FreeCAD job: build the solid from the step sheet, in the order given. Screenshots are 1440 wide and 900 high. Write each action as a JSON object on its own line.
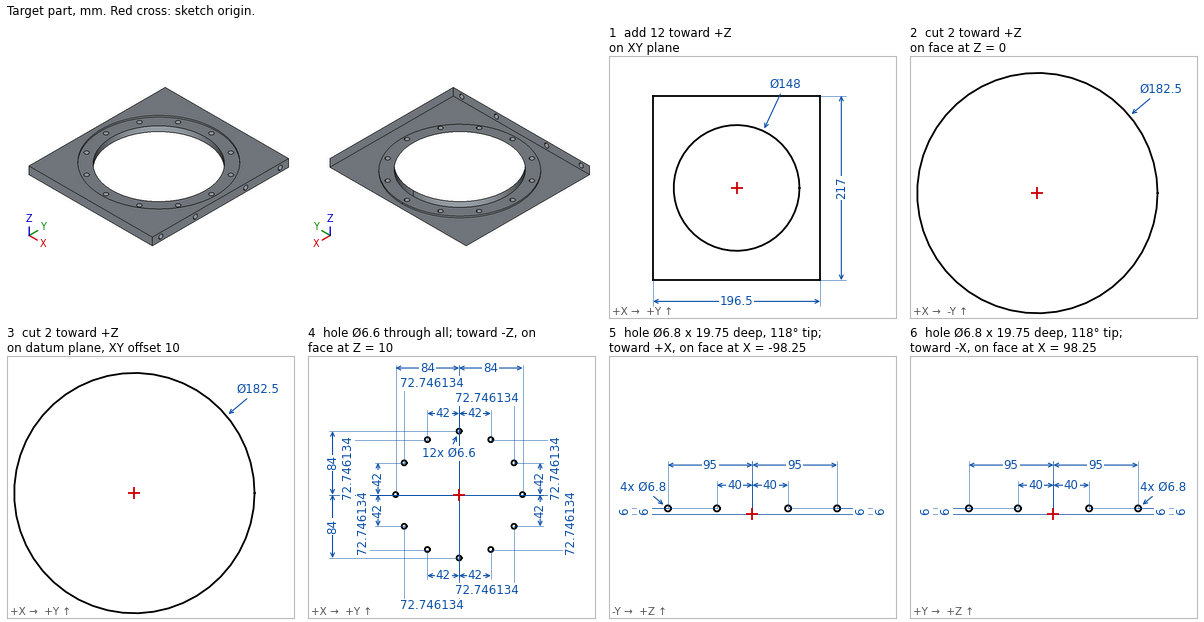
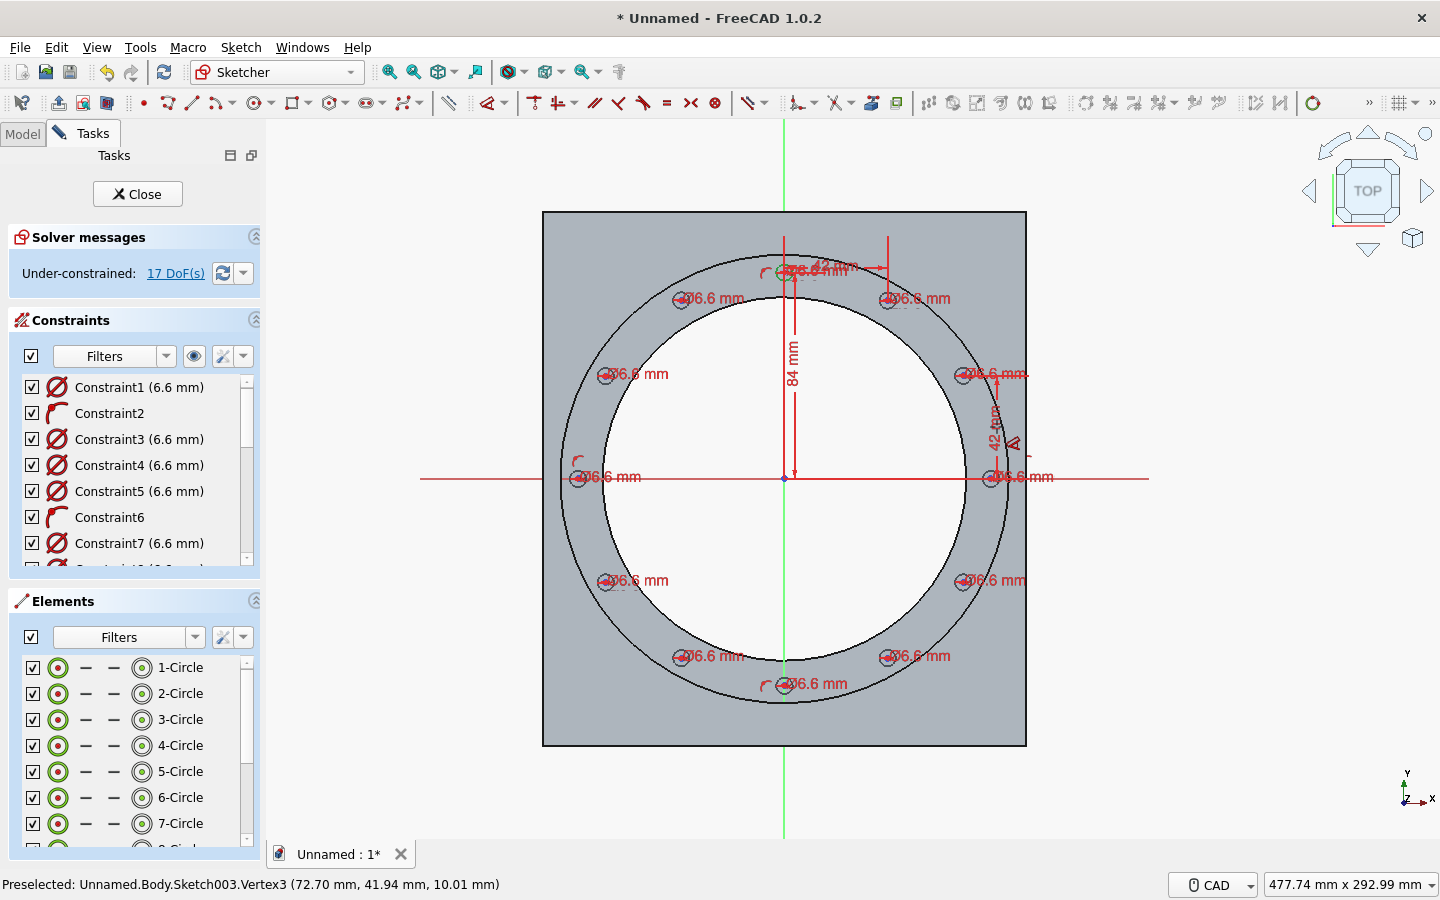
{"action": "left_click", "coordinate": [991, 479]}
{"action": "left_click", "coordinate": [888, 513]}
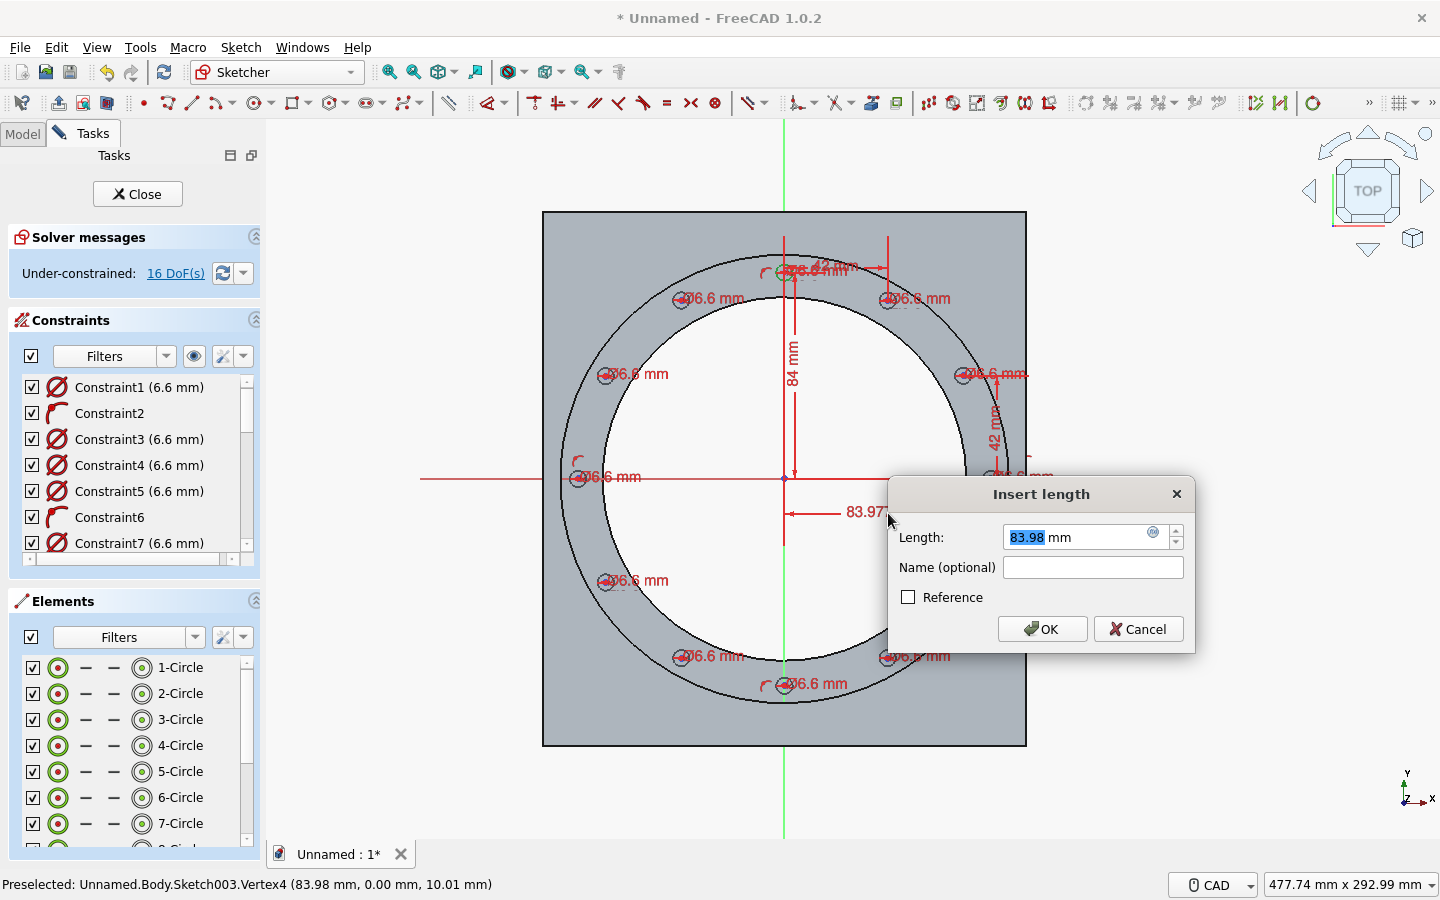
{"action": "type", "text": "84"}
{"action": "key", "text": "Return"}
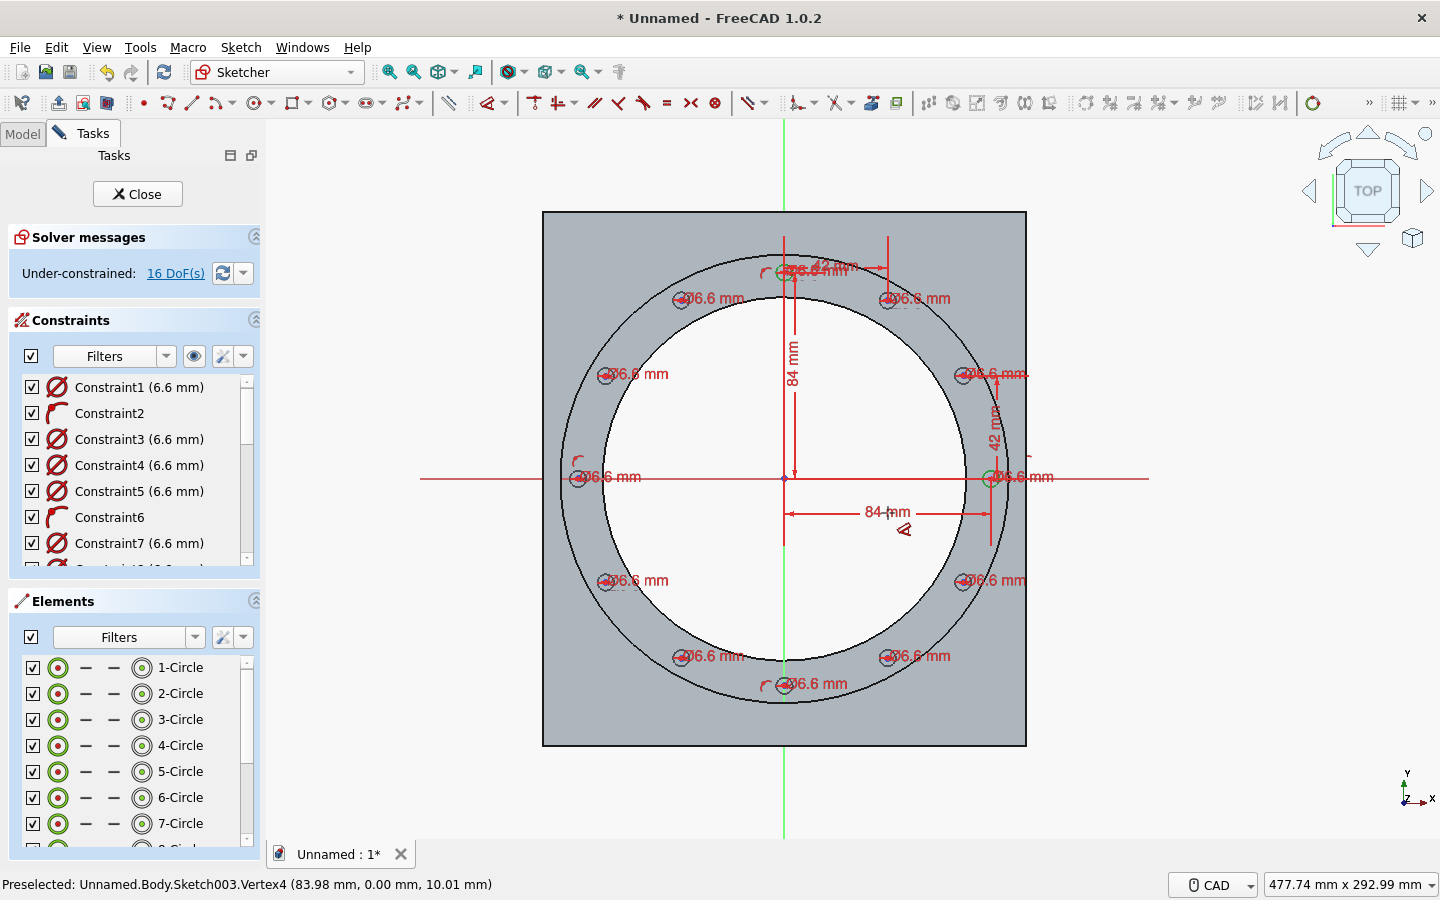
{"action": "left_click", "coordinate": [963, 582]}
{"action": "left_click", "coordinate": [997, 531]}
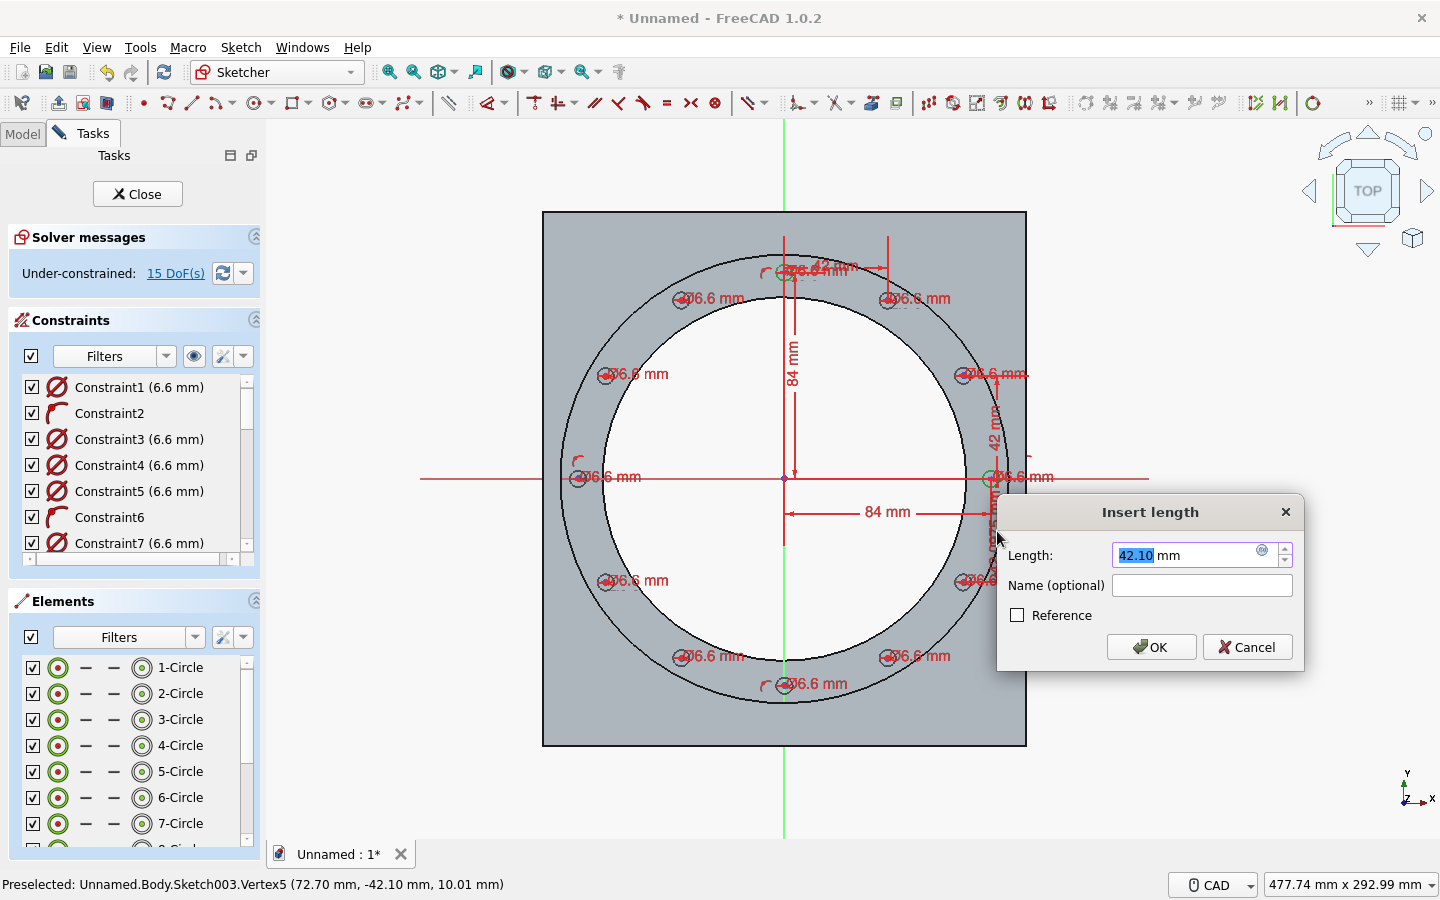
{"action": "type", "text": "42"}
{"action": "key", "text": "Return"}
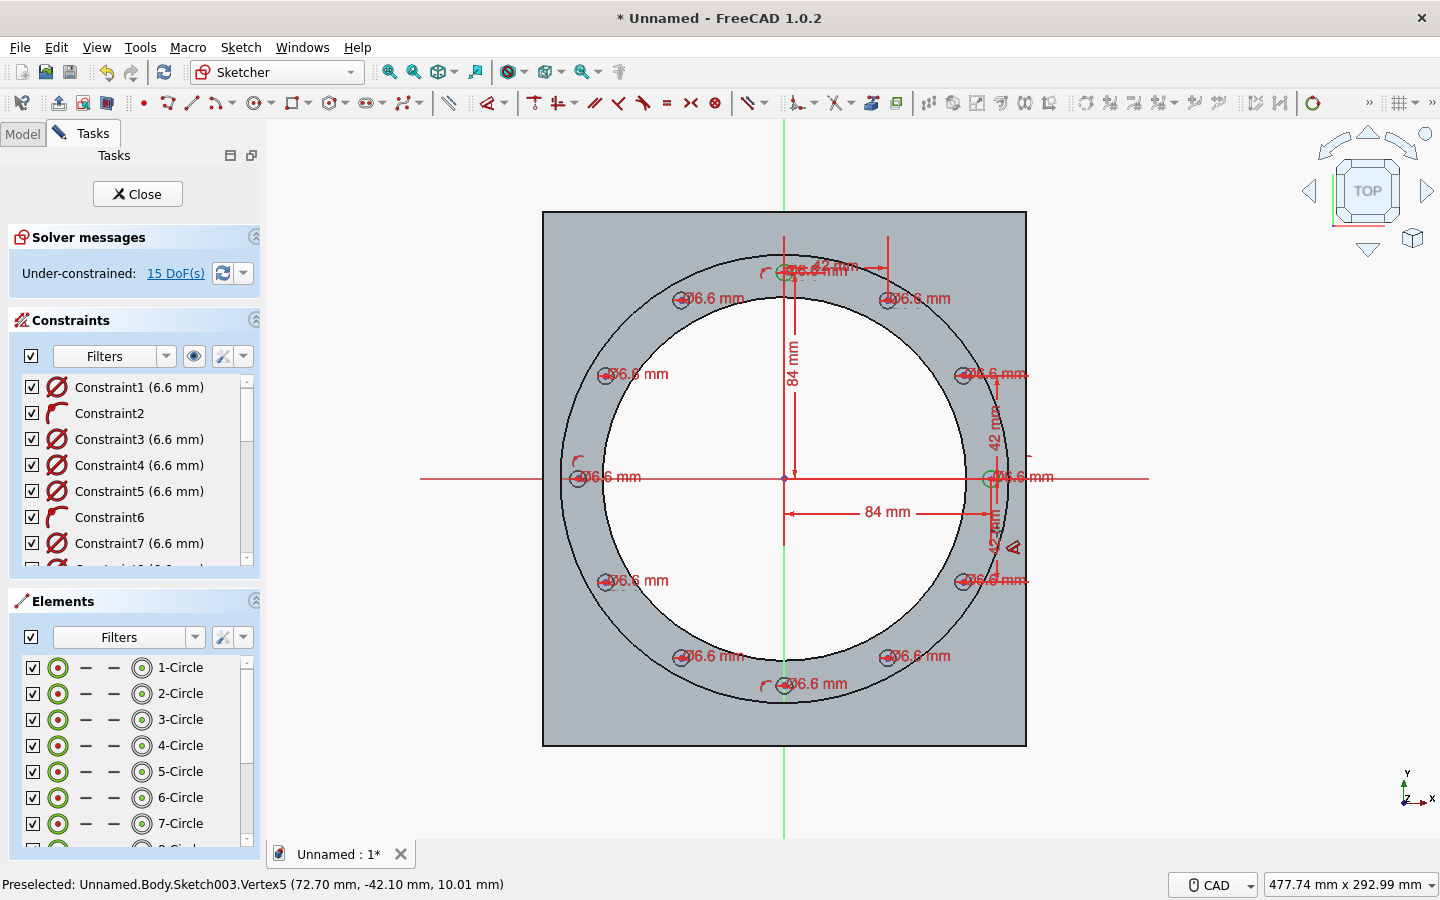
{"action": "left_click", "coordinate": [888, 658]}
{"action": "left_click", "coordinate": [836, 692]}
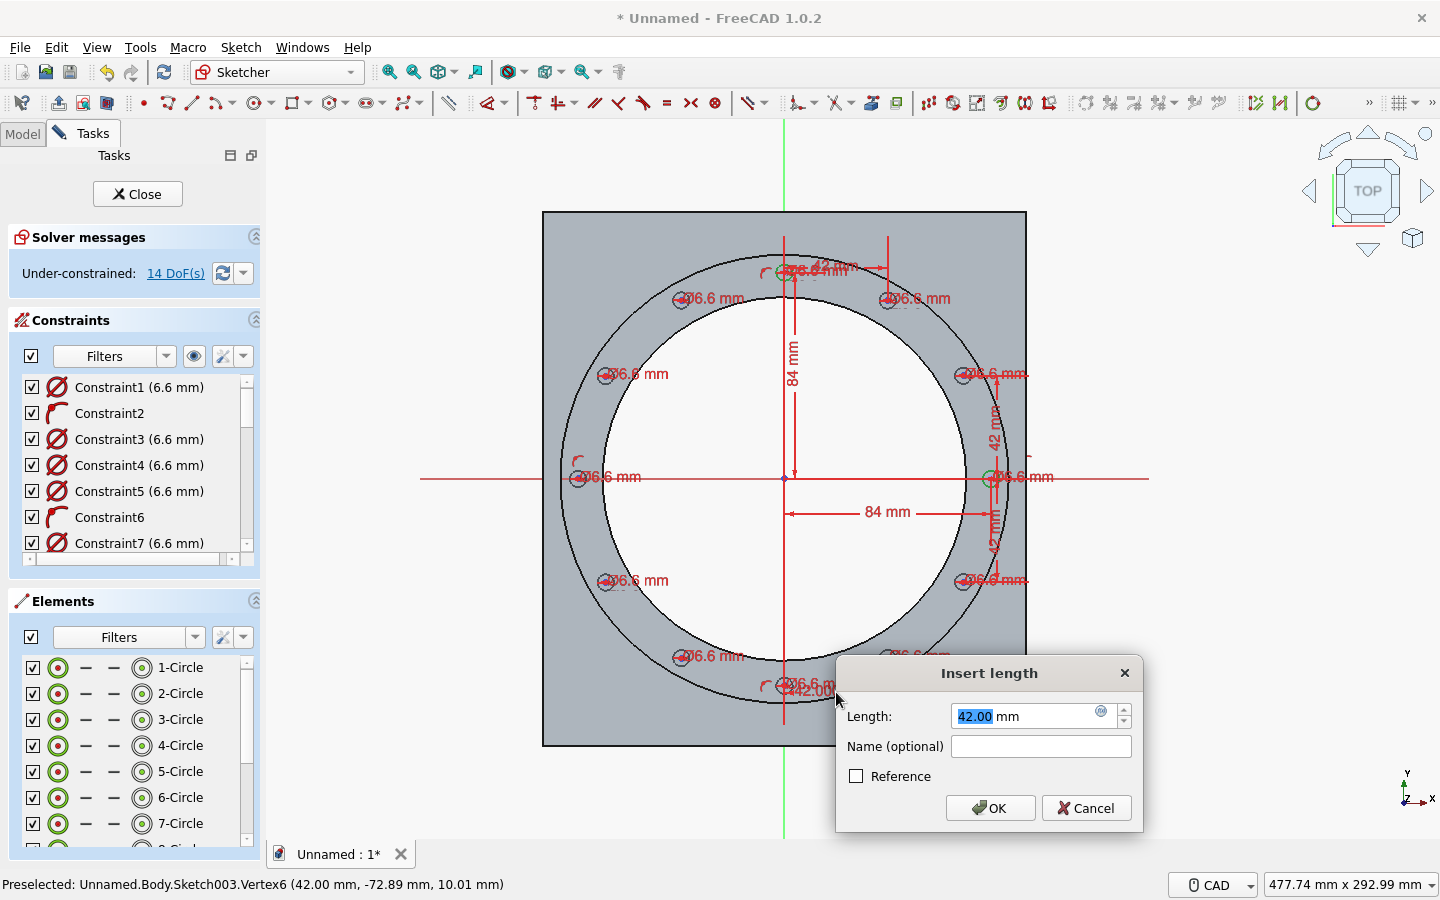
{"action": "type", "text": "42"}
{"action": "key", "text": "Return"}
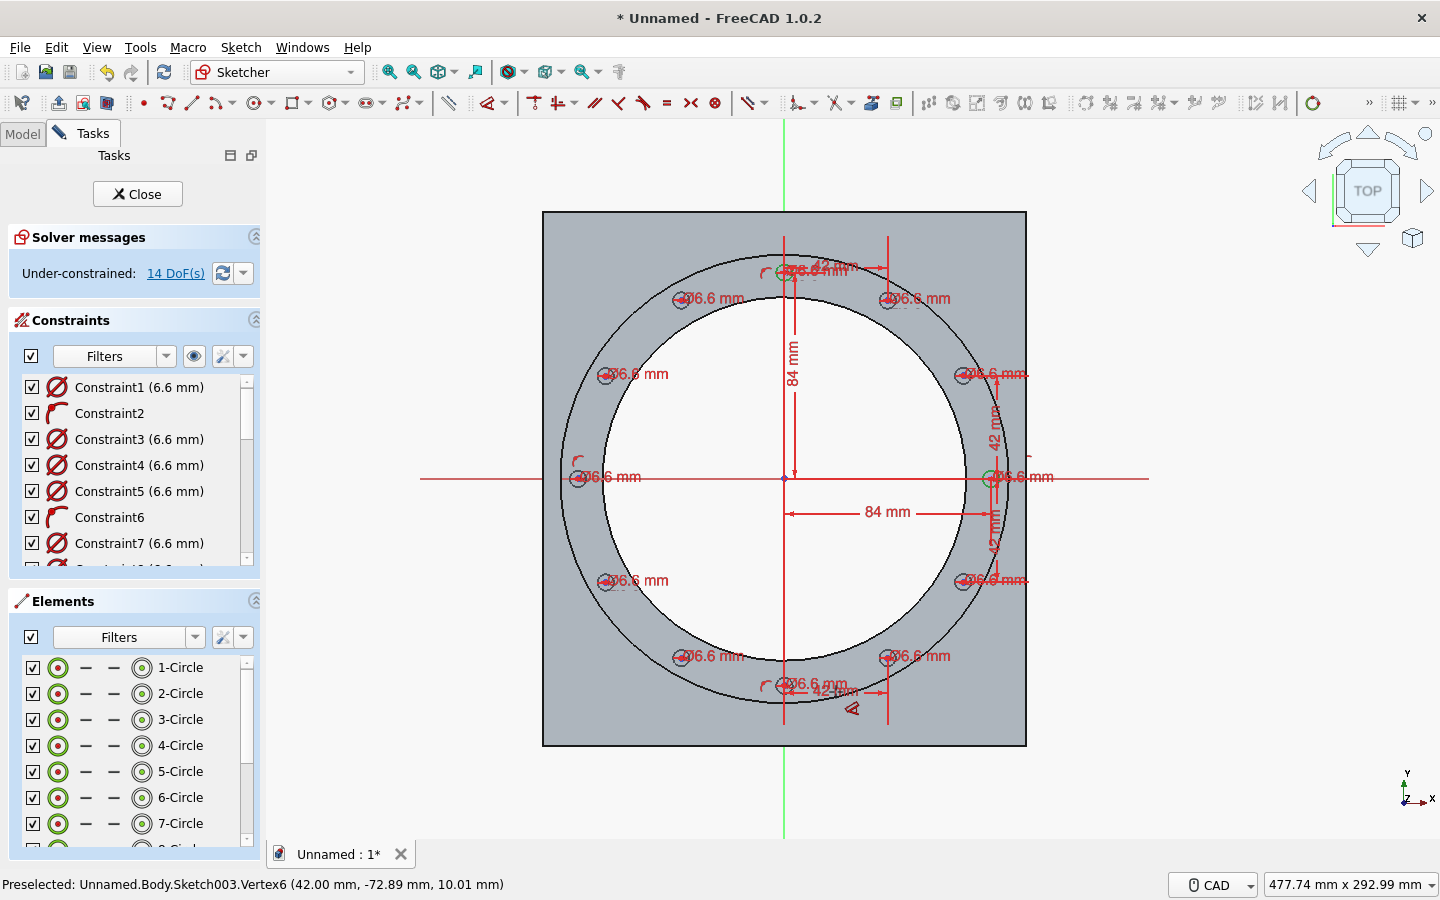
{"action": "left_click", "coordinate": [784, 686]}
{"action": "left_click", "coordinate": [818, 582]}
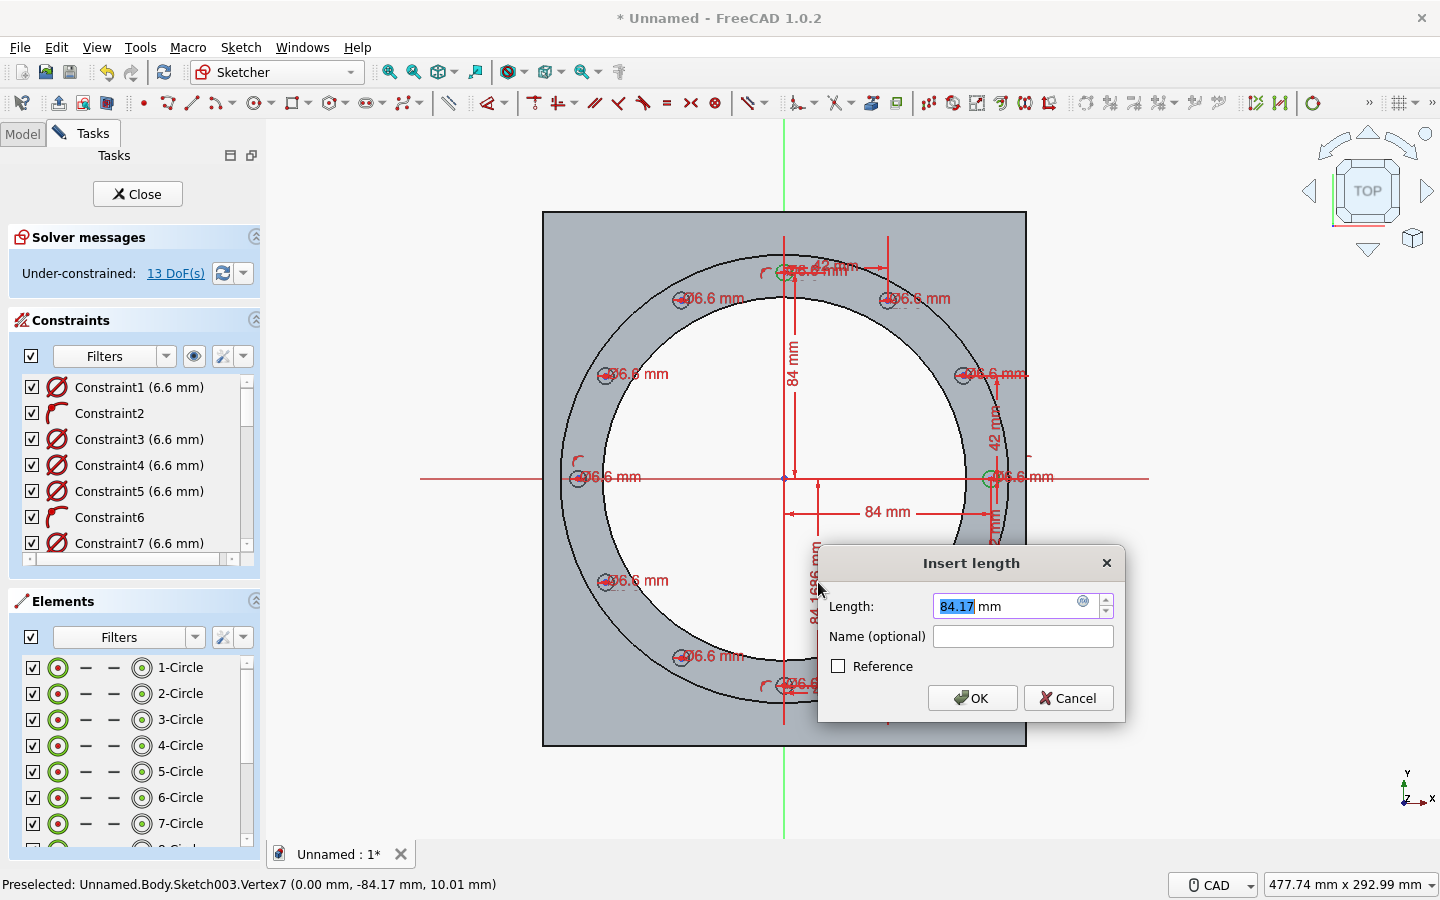
{"action": "type", "text": "84"}
{"action": "key", "text": "Return"}